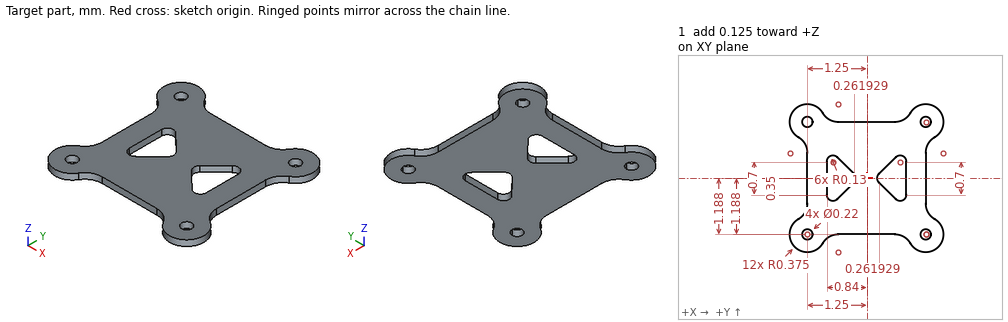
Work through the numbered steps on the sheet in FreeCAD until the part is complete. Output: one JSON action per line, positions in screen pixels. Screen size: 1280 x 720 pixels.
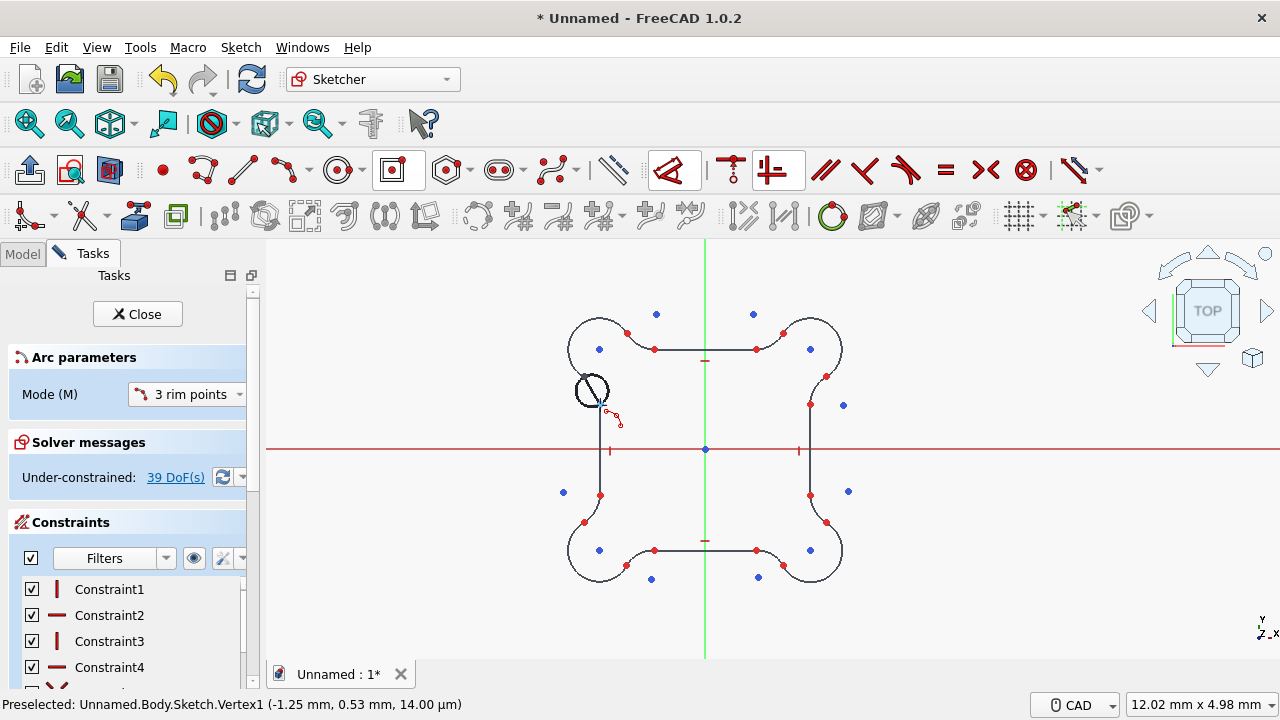
{"action": "scroll", "coordinate": [595, 388], "scroll_direction": "up", "scroll_amount": 7}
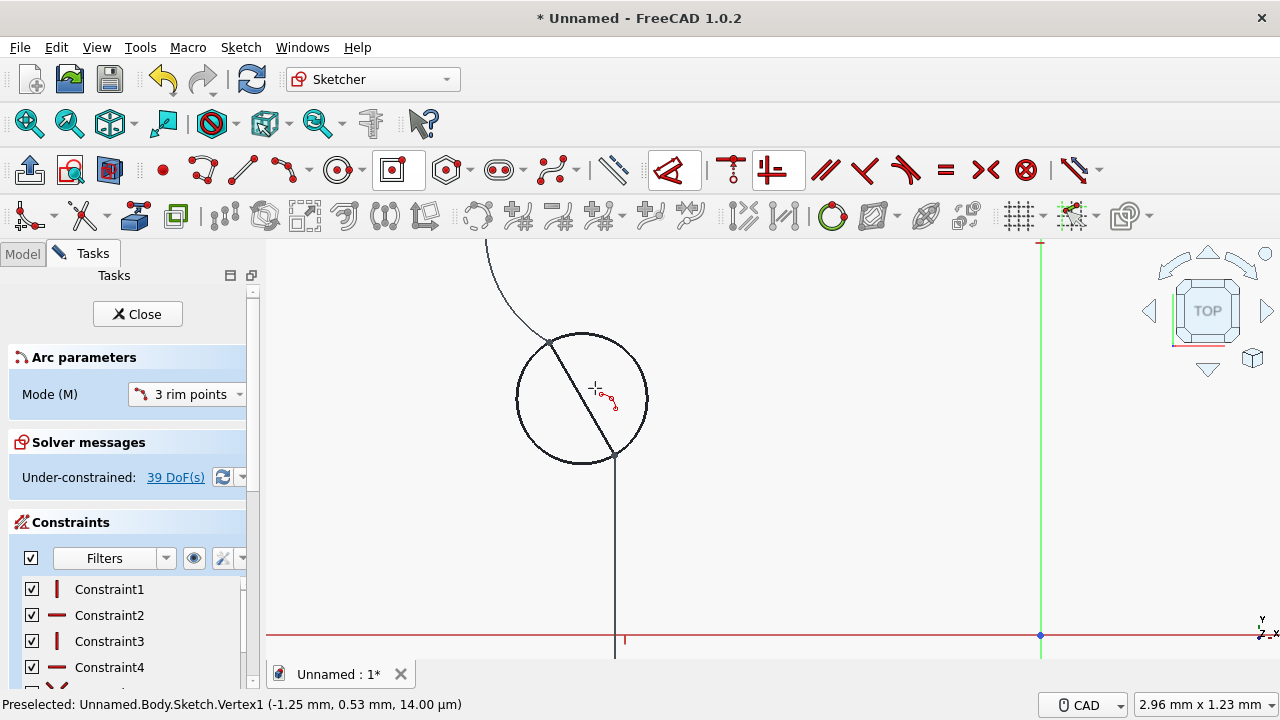
{"action": "left_click", "coordinate": [596, 387]}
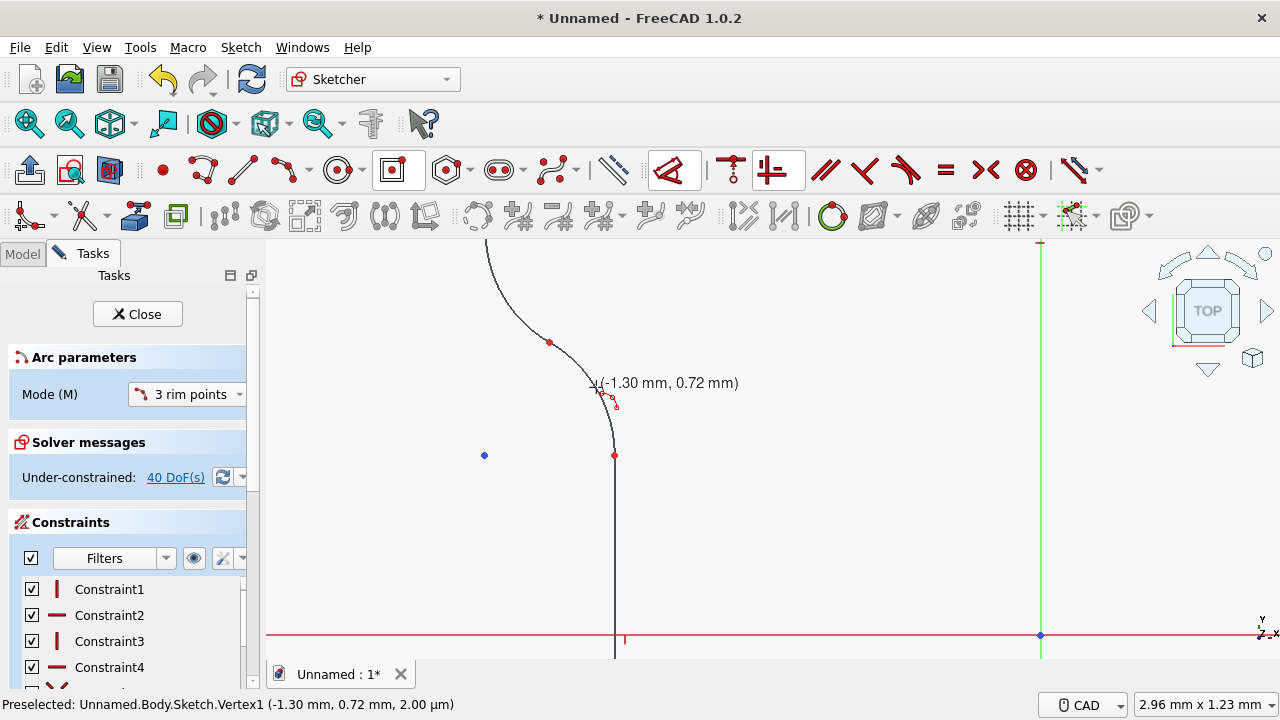
{"action": "left_click", "coordinate": [244, 170]}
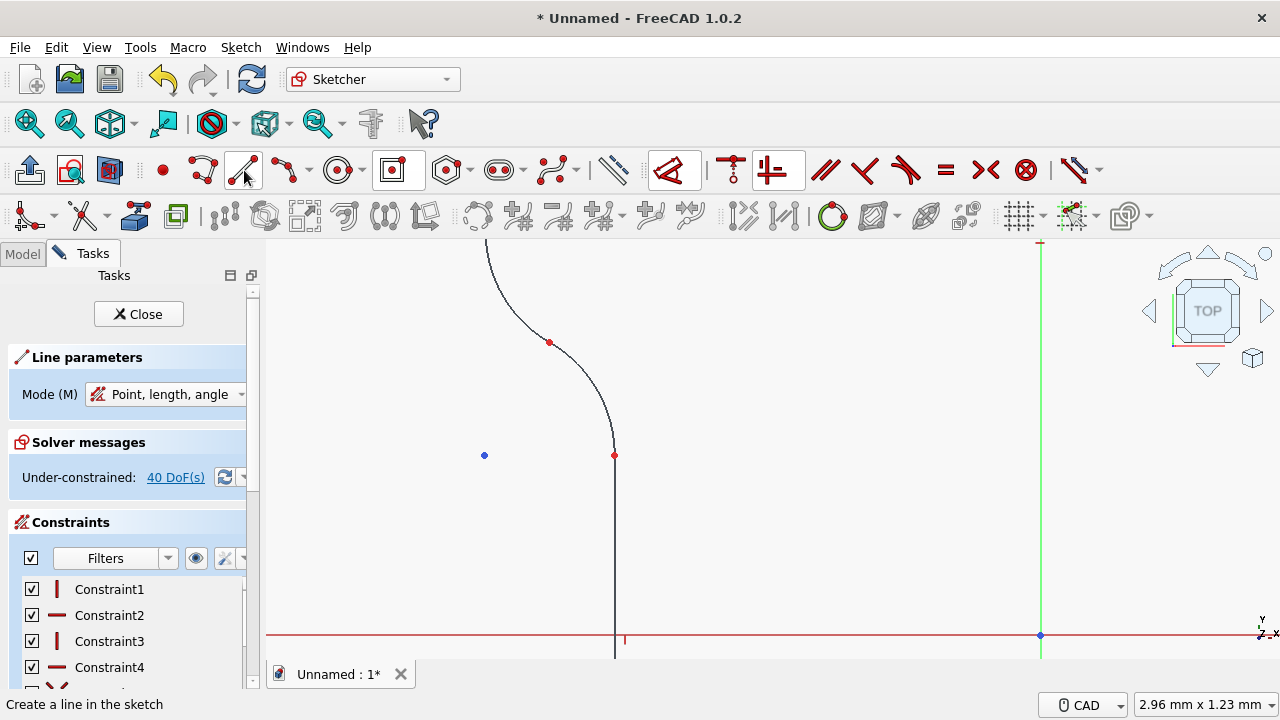
{"action": "scroll", "coordinate": [594, 388], "scroll_direction": "down", "scroll_amount": 7}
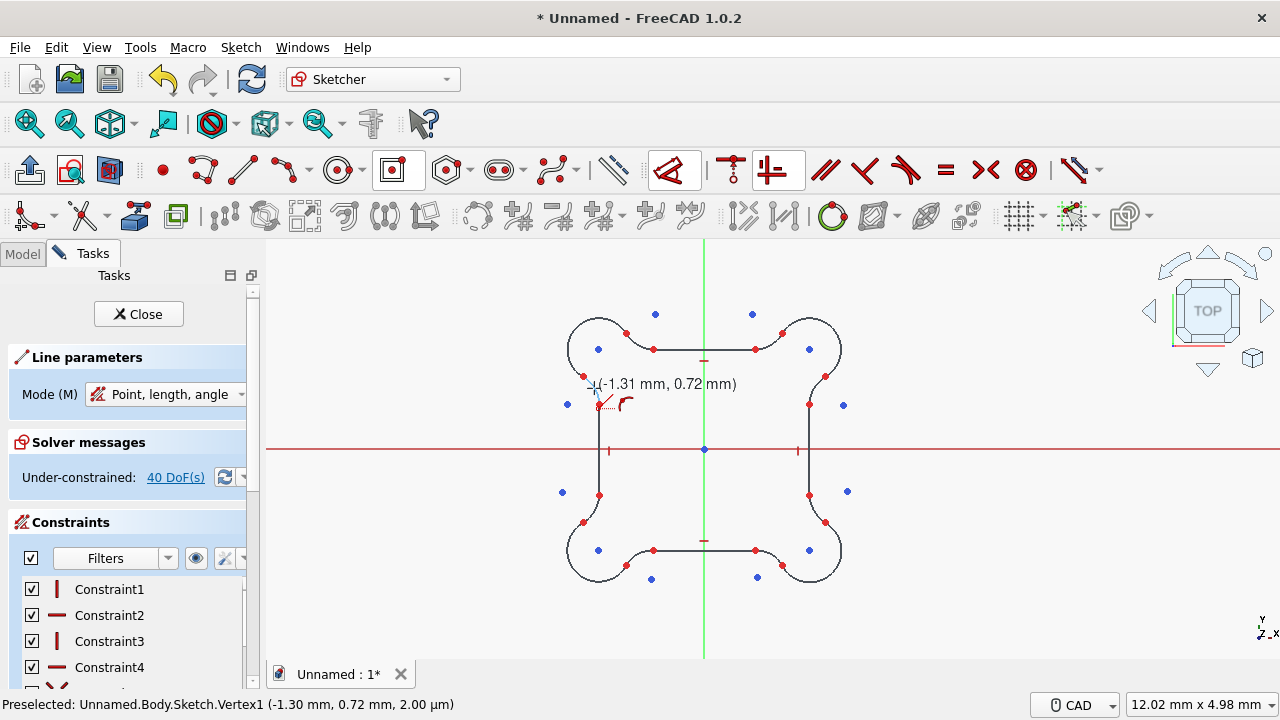
{"action": "left_click", "coordinate": [634, 479]}
{"action": "left_click", "coordinate": [634, 420]}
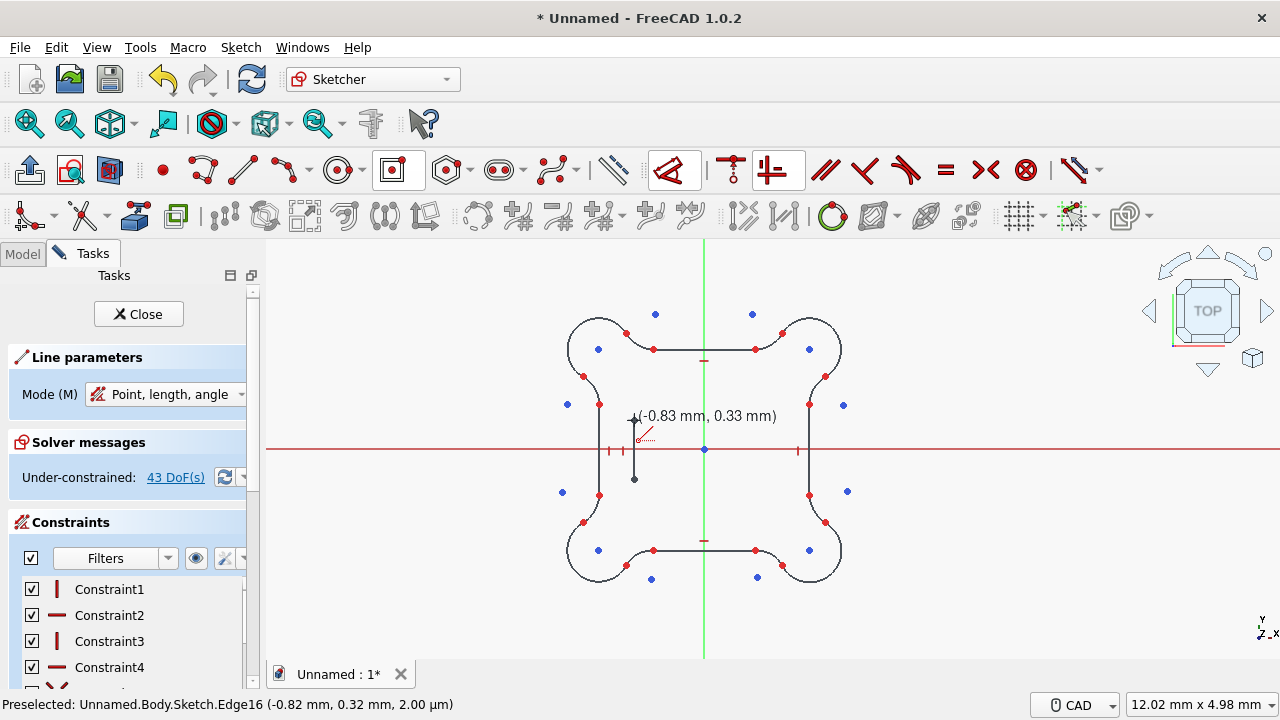
{"action": "left_click", "coordinate": [652, 412]}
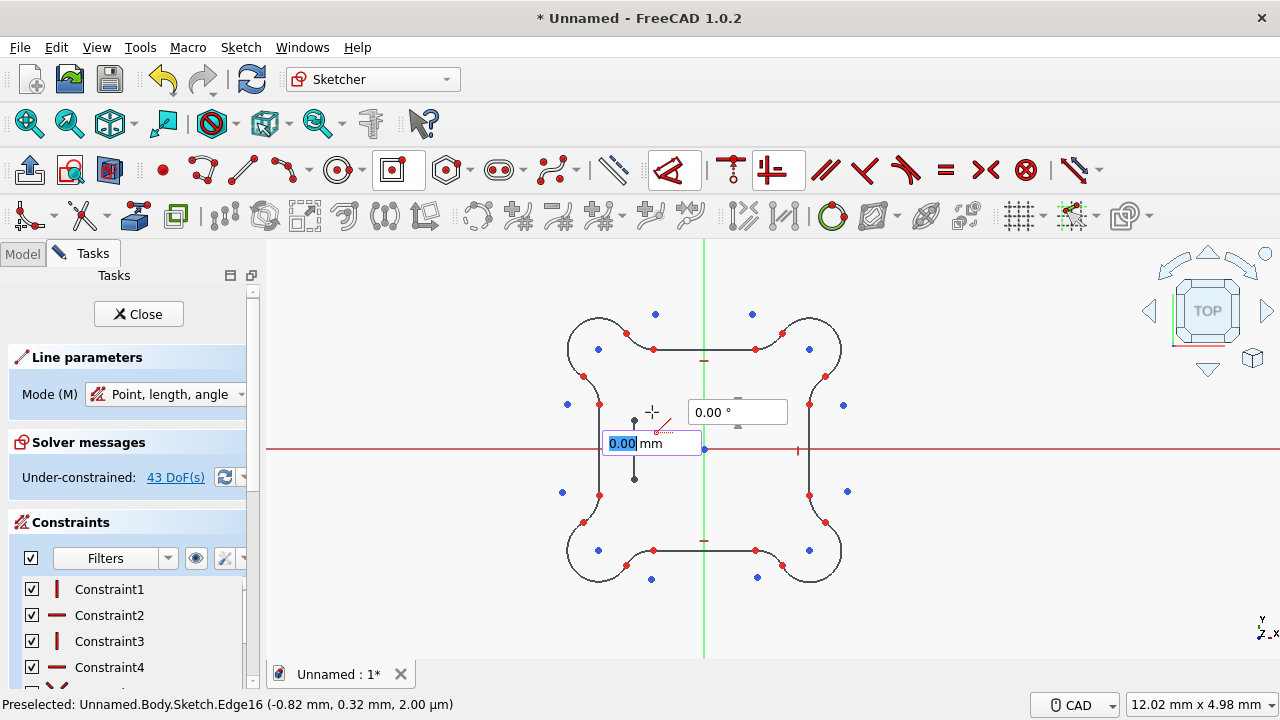
{"action": "scroll", "coordinate": [682, 441], "scroll_direction": "up", "scroll_amount": 4}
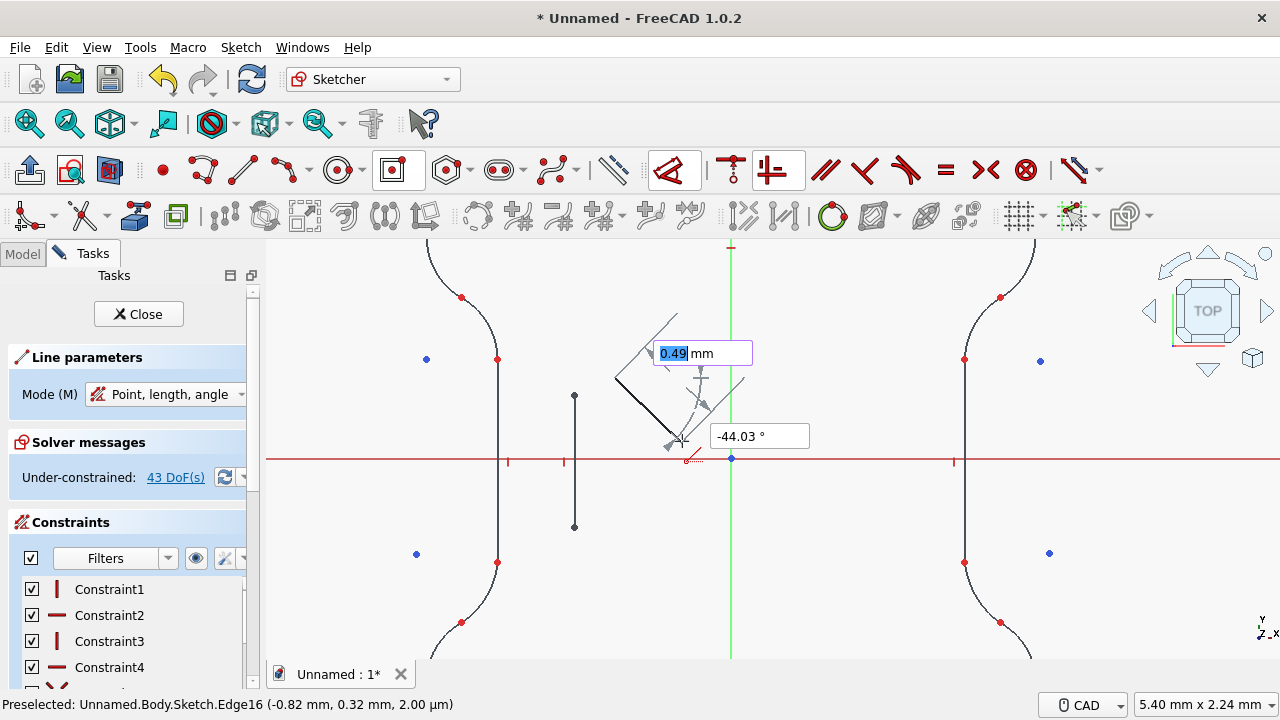
{"action": "left_click", "coordinate": [682, 441]}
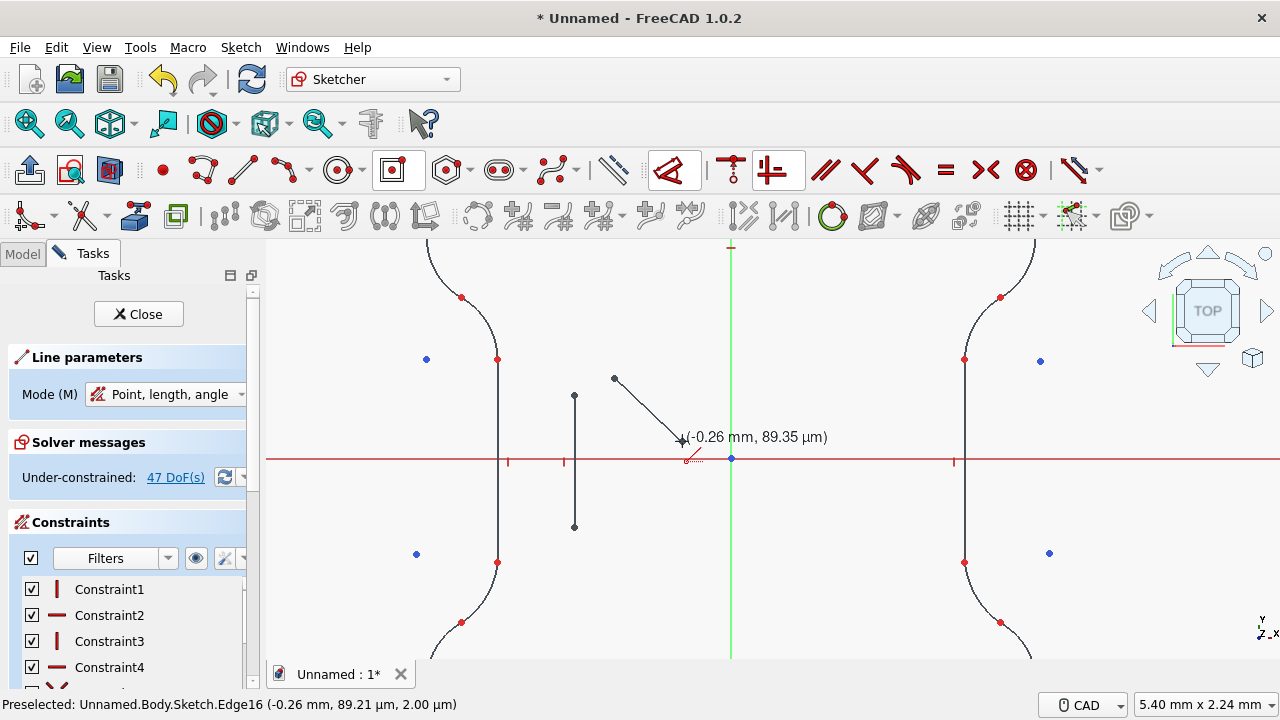
{"action": "left_click", "coordinate": [682, 476]}
{"action": "left_click", "coordinate": [615, 542]}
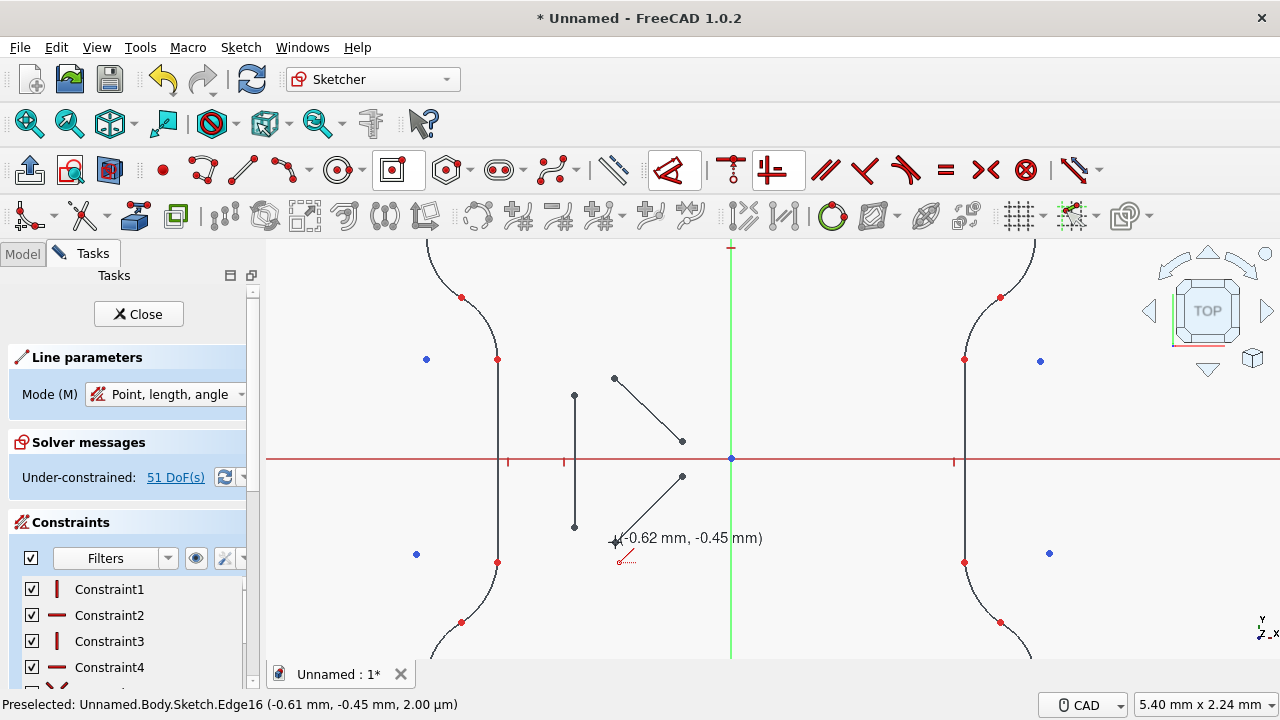
{"action": "left_click", "coordinate": [284, 170]}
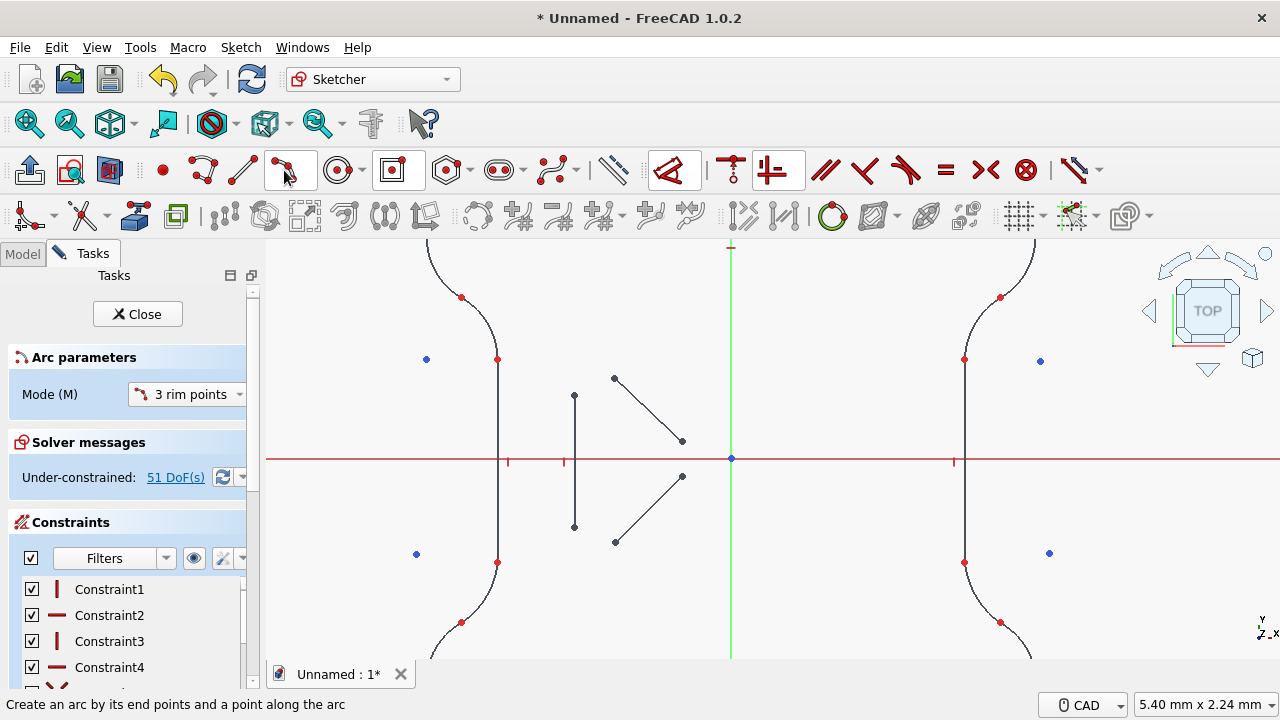
{"action": "left_click", "coordinate": [575, 396]}
{"action": "left_click", "coordinate": [615, 378]}
{"action": "left_click", "coordinate": [589, 371]}